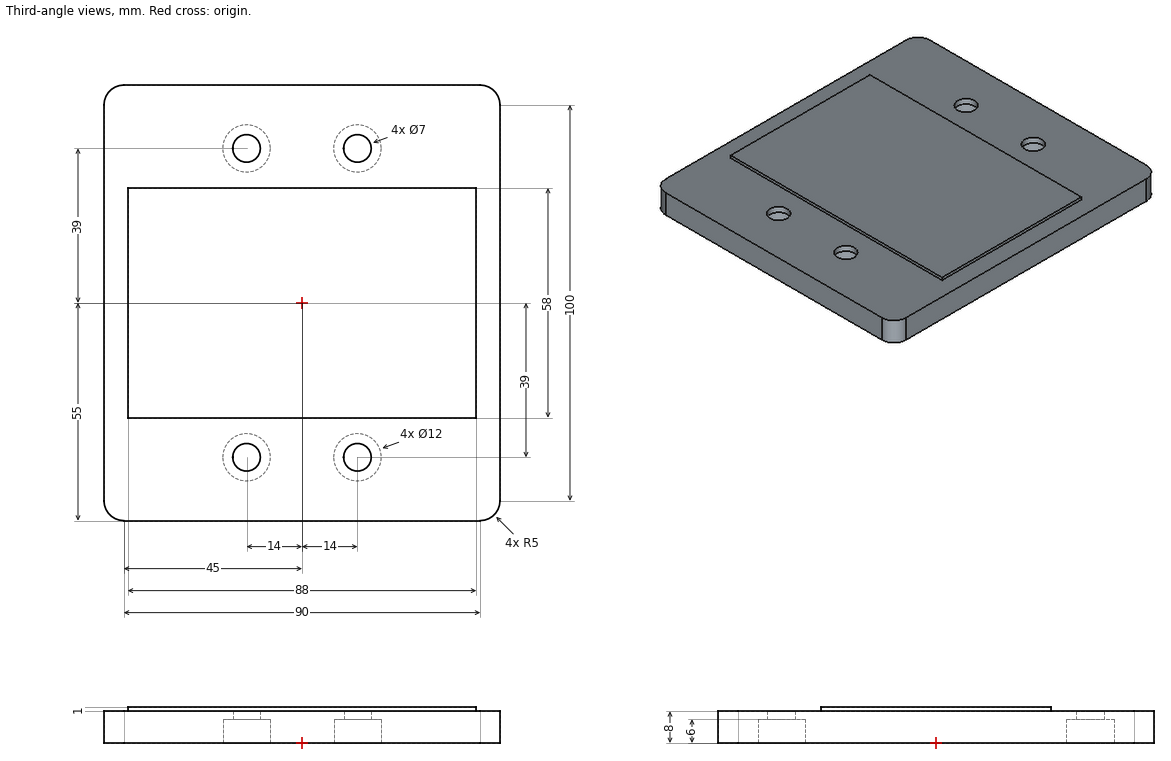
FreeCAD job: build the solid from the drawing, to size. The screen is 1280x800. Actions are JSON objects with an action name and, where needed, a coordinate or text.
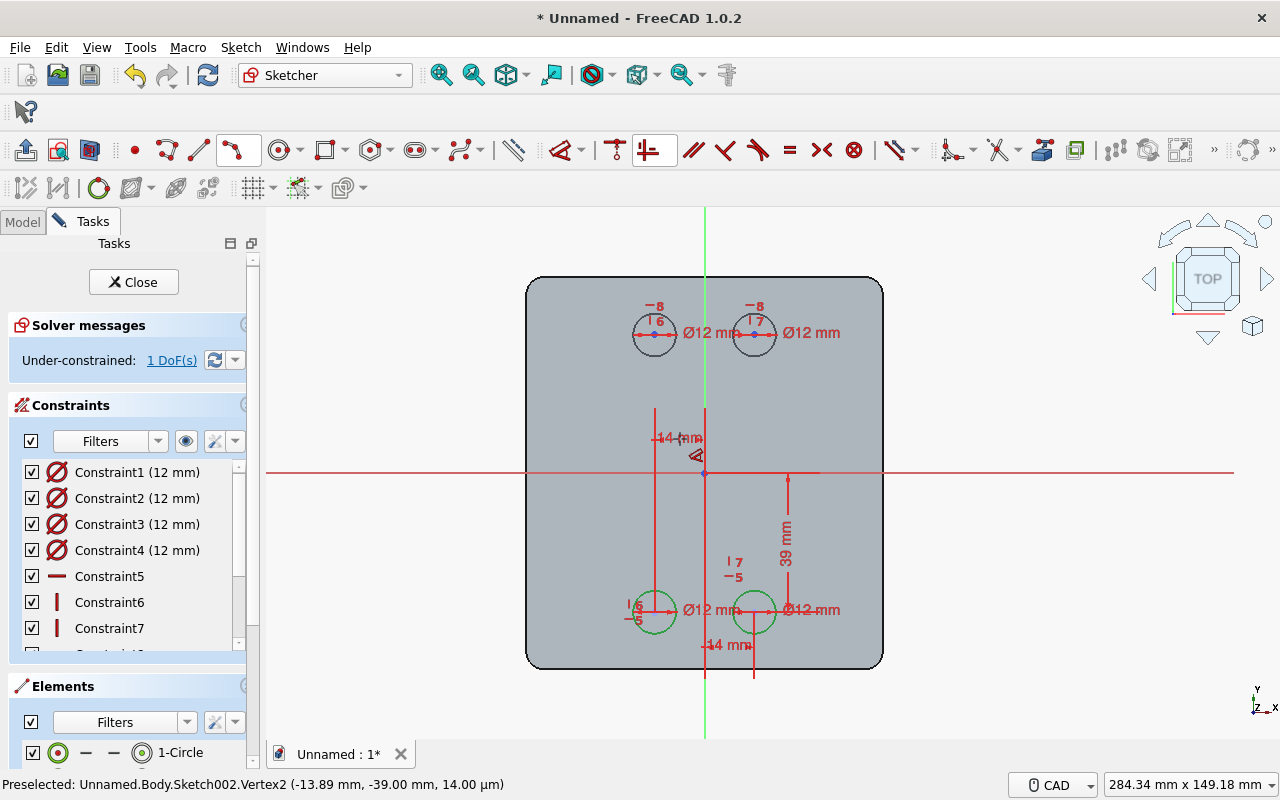
{"action": "left_click", "coordinate": [655, 335]}
{"action": "left_click", "coordinate": [621, 404]}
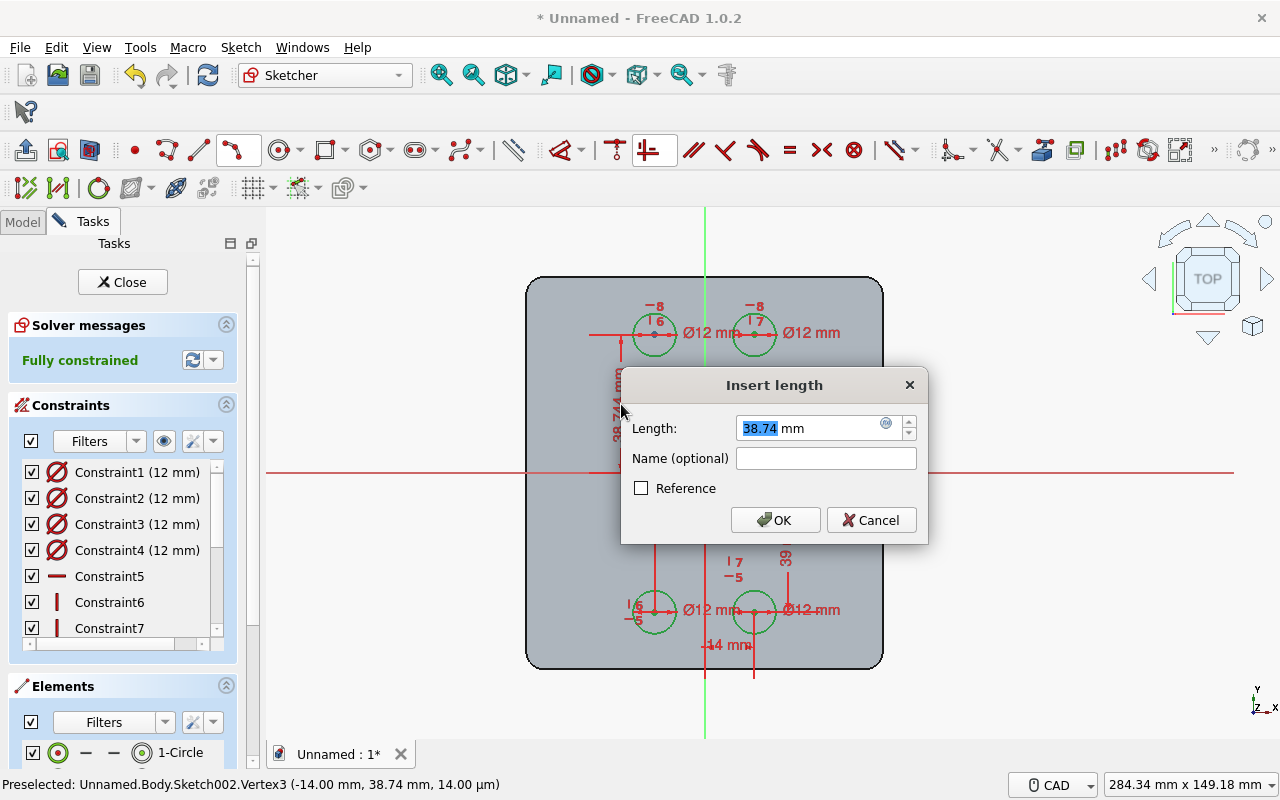
{"action": "type", "text": "39"}
{"action": "key", "text": "Return"}
{"action": "key", "text": "Escape"}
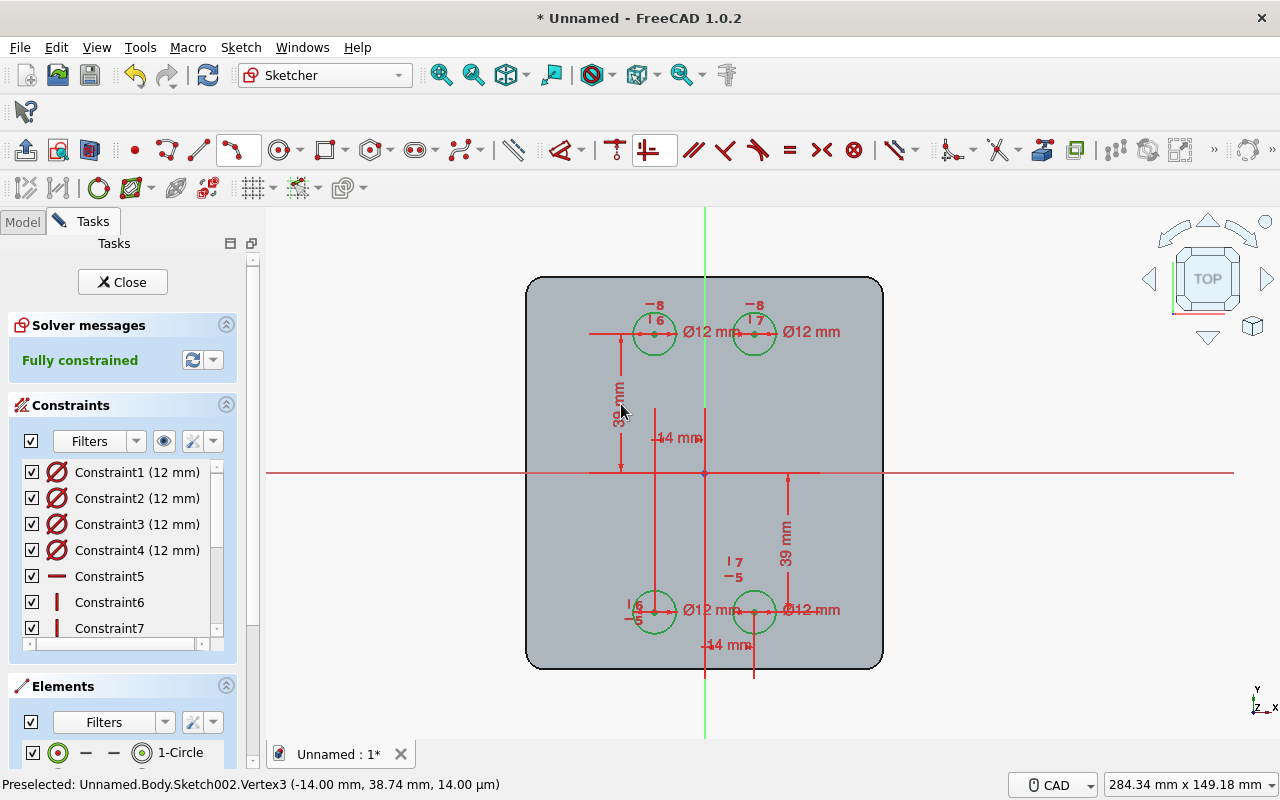
{"action": "left_click", "coordinate": [123, 282]}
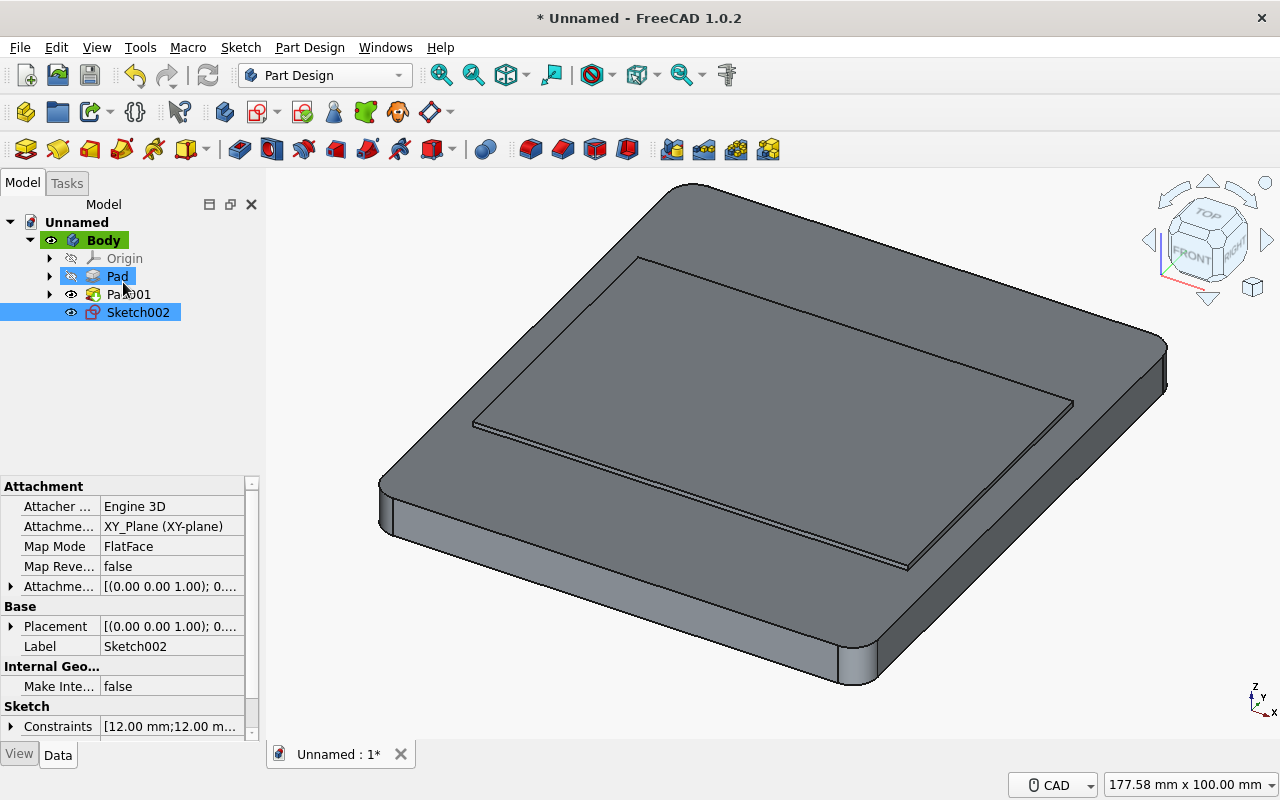
{"action": "left_click", "coordinate": [240, 150]}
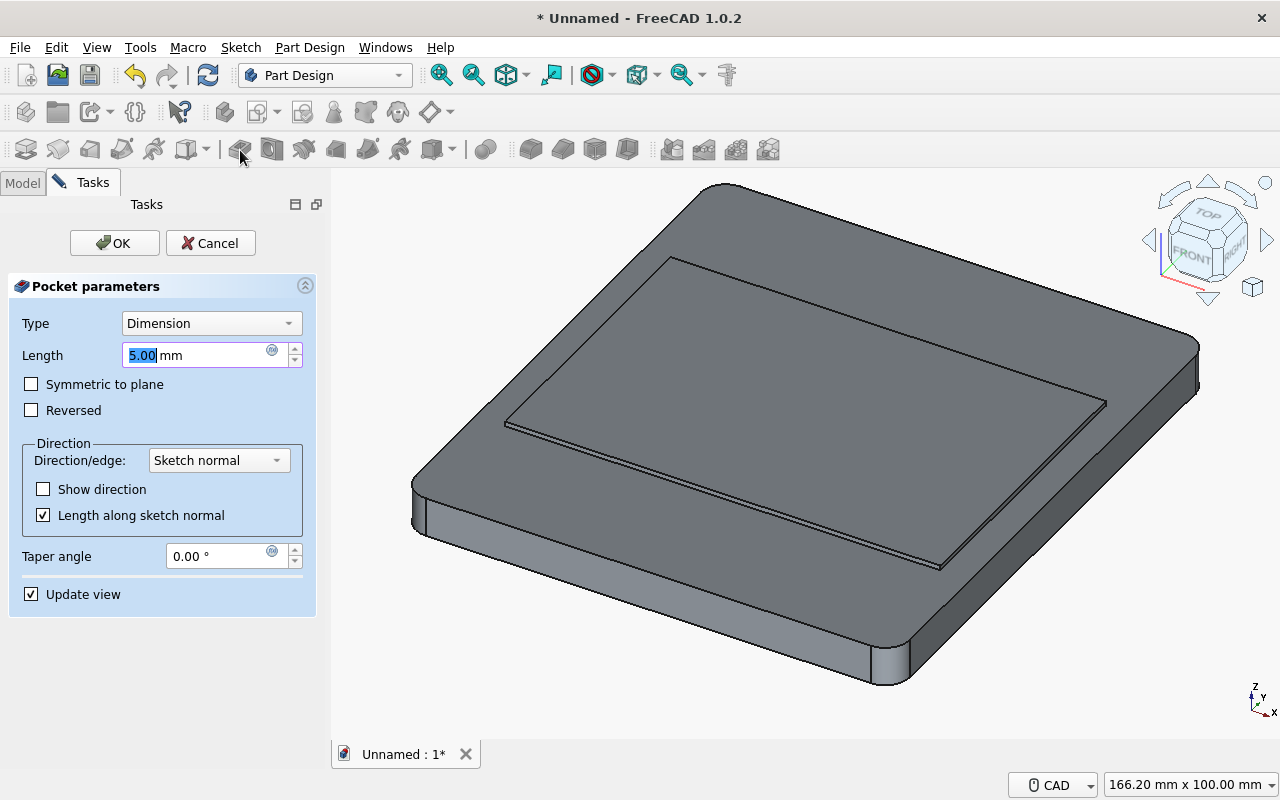
{"action": "type", "text": "6"}
{"action": "key", "text": "Tab"}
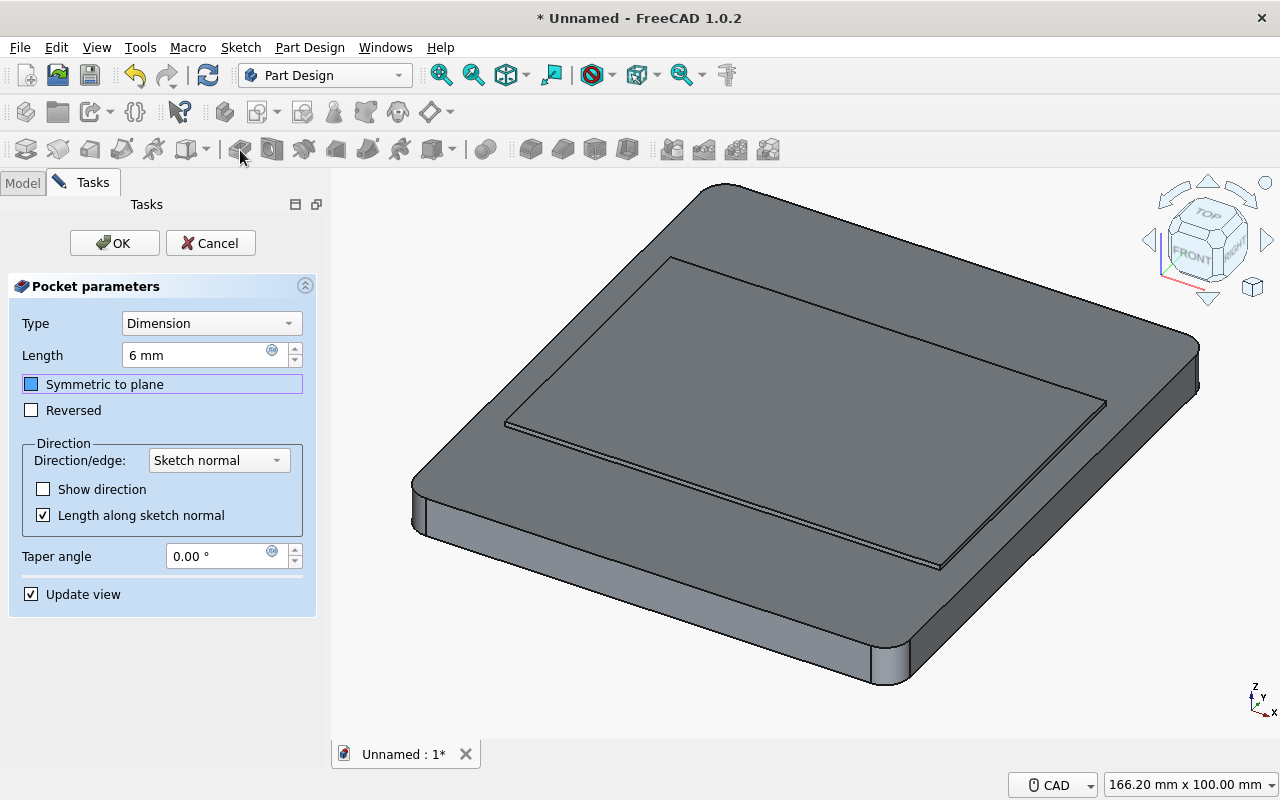
{"action": "left_click", "coordinate": [30, 410]}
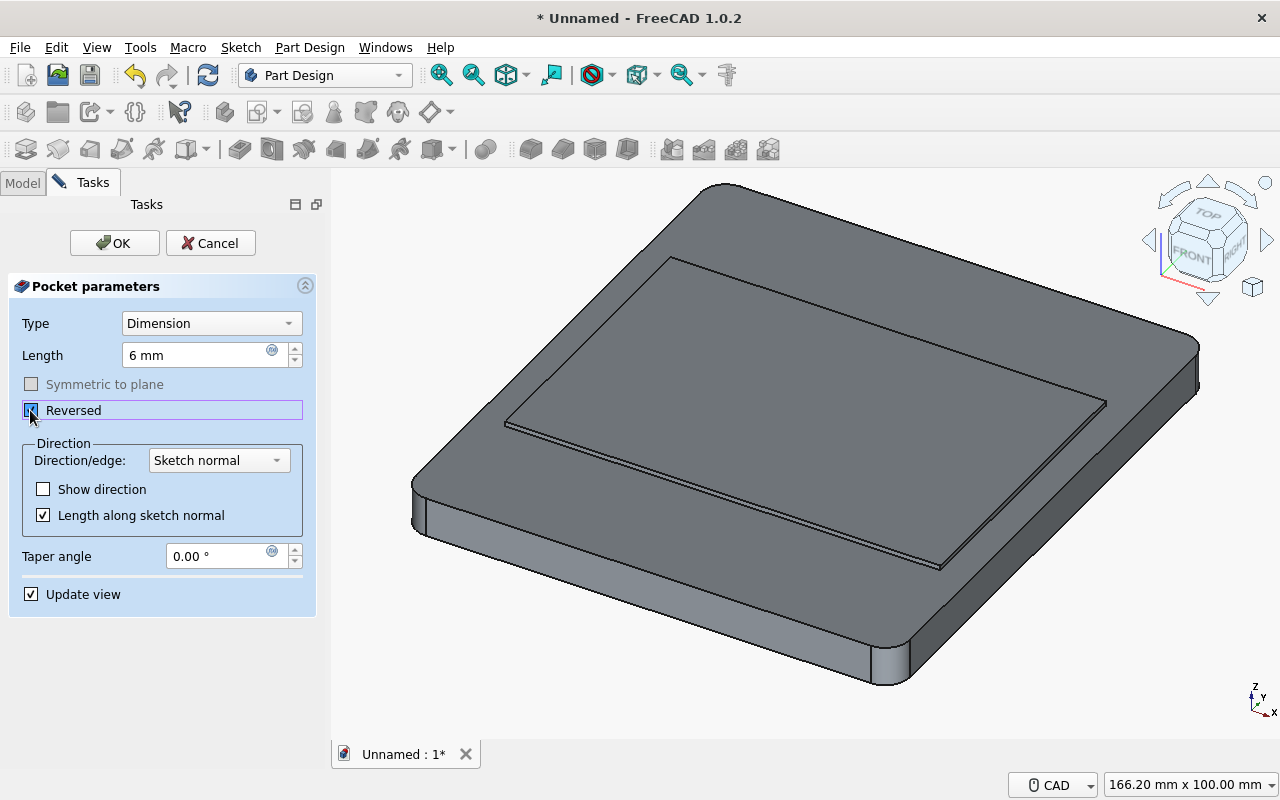
{"action": "left_click", "coordinate": [115, 243]}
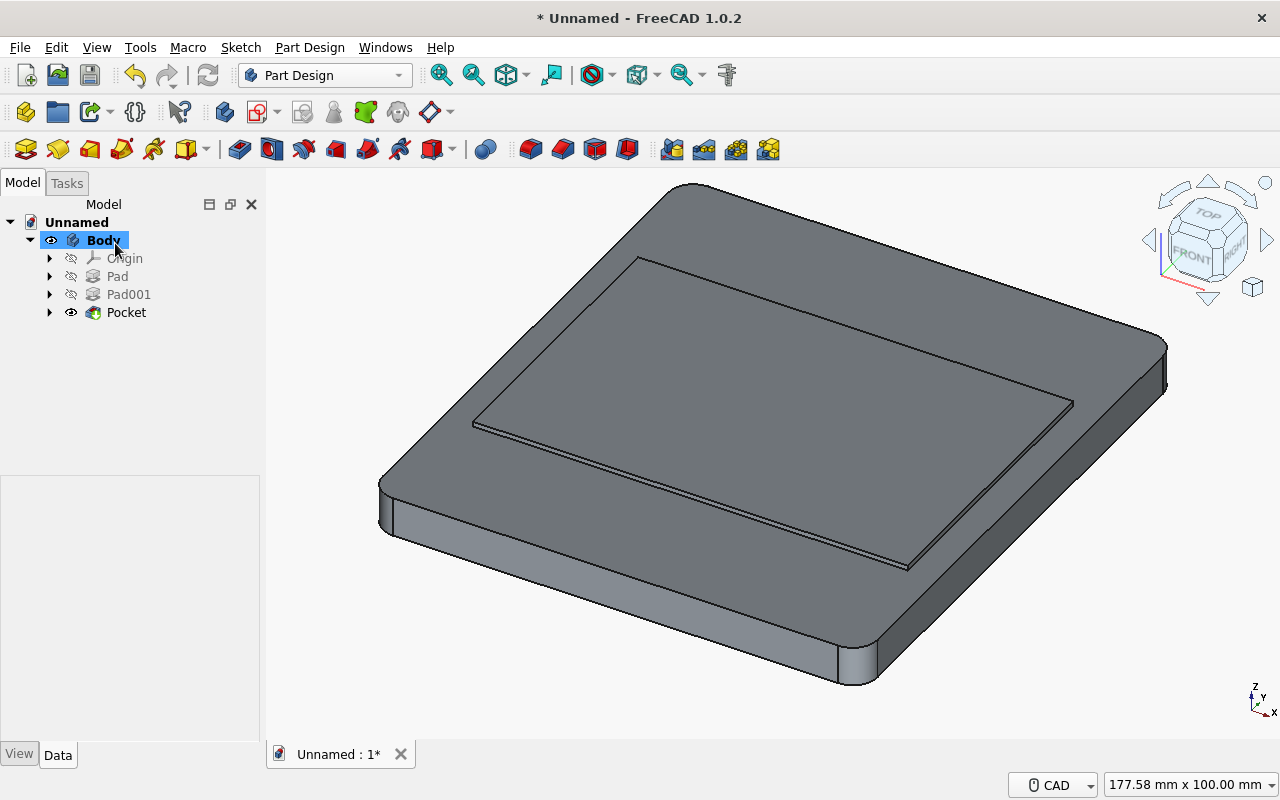
{"action": "key", "text": "5"}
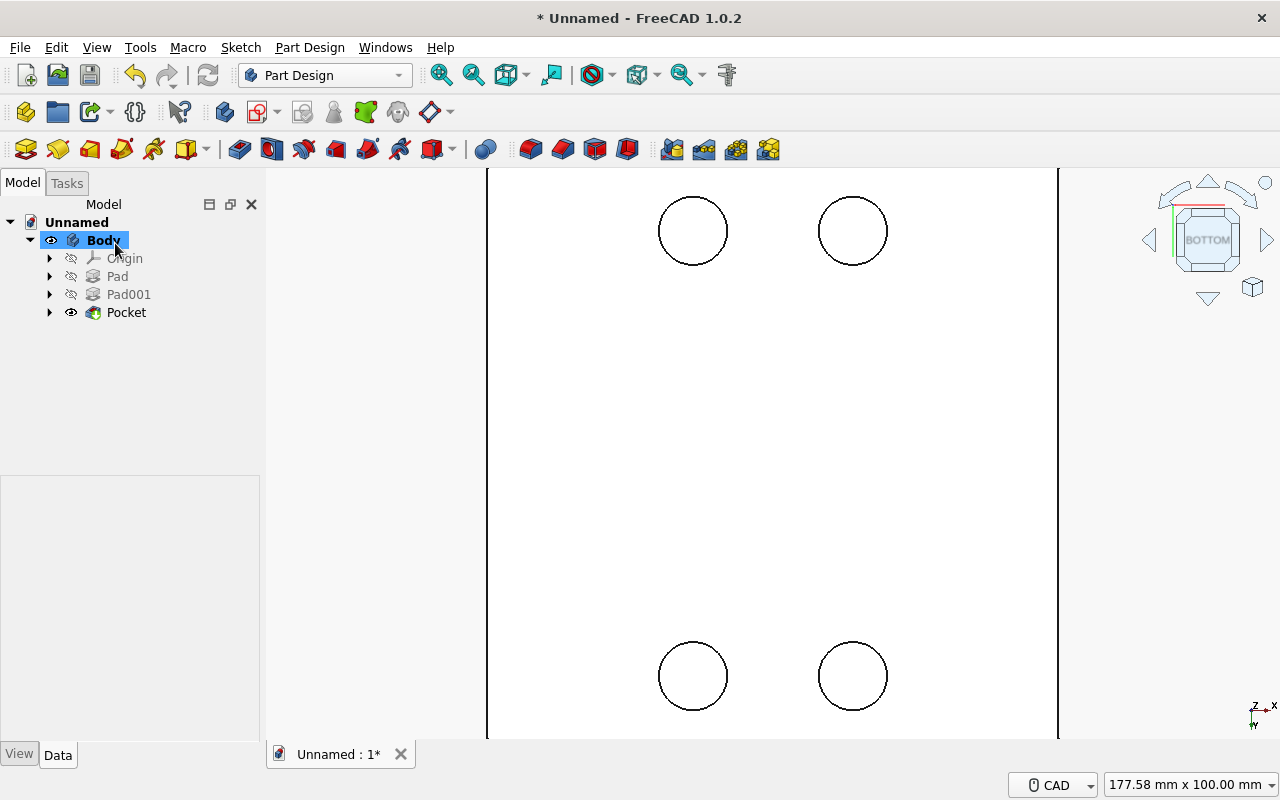
{"action": "key", "text": "v f"}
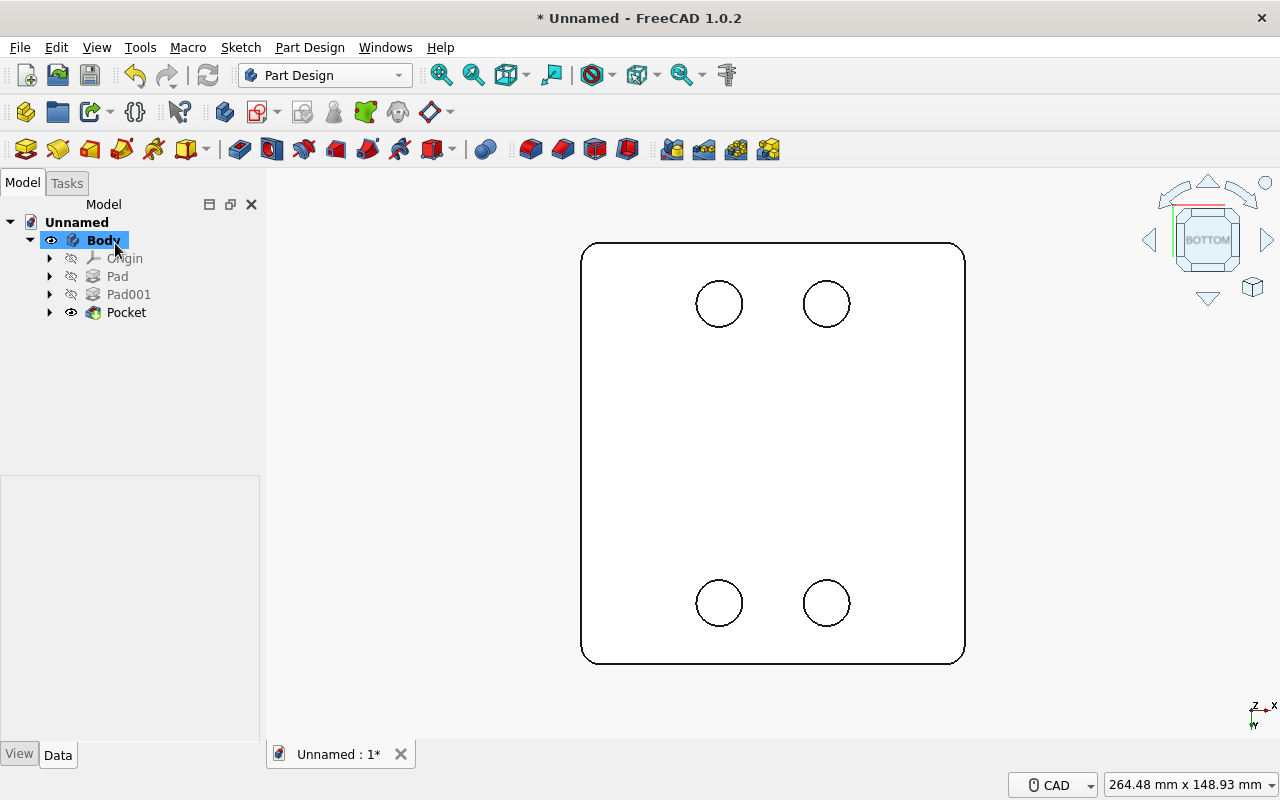
{"action": "left_click", "coordinate": [827, 602]}